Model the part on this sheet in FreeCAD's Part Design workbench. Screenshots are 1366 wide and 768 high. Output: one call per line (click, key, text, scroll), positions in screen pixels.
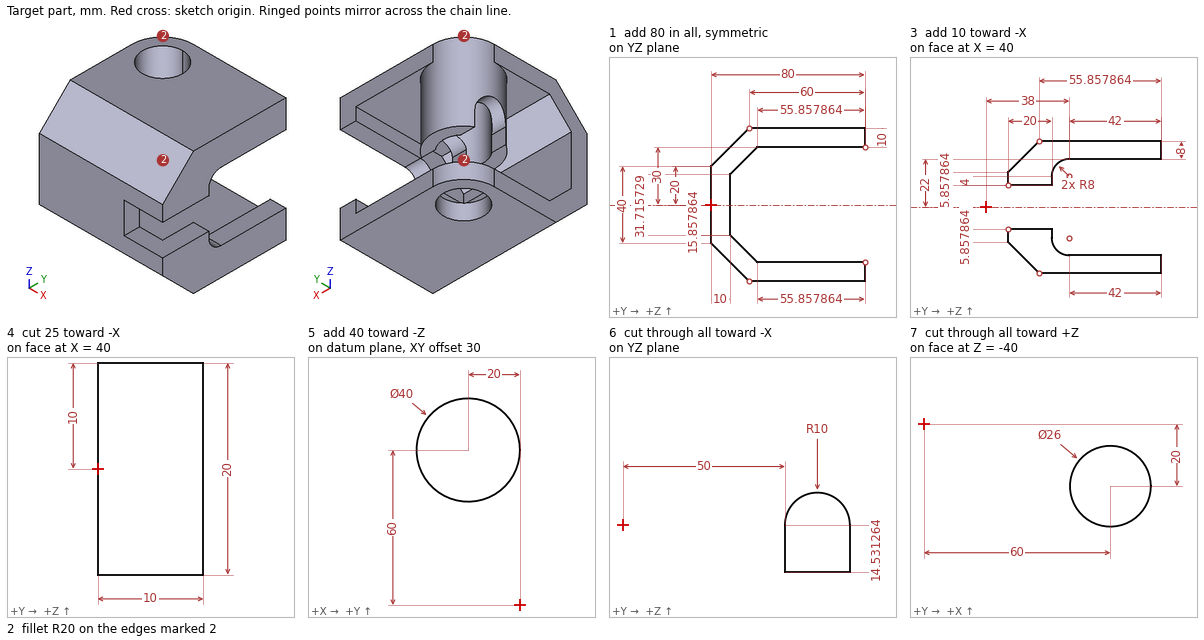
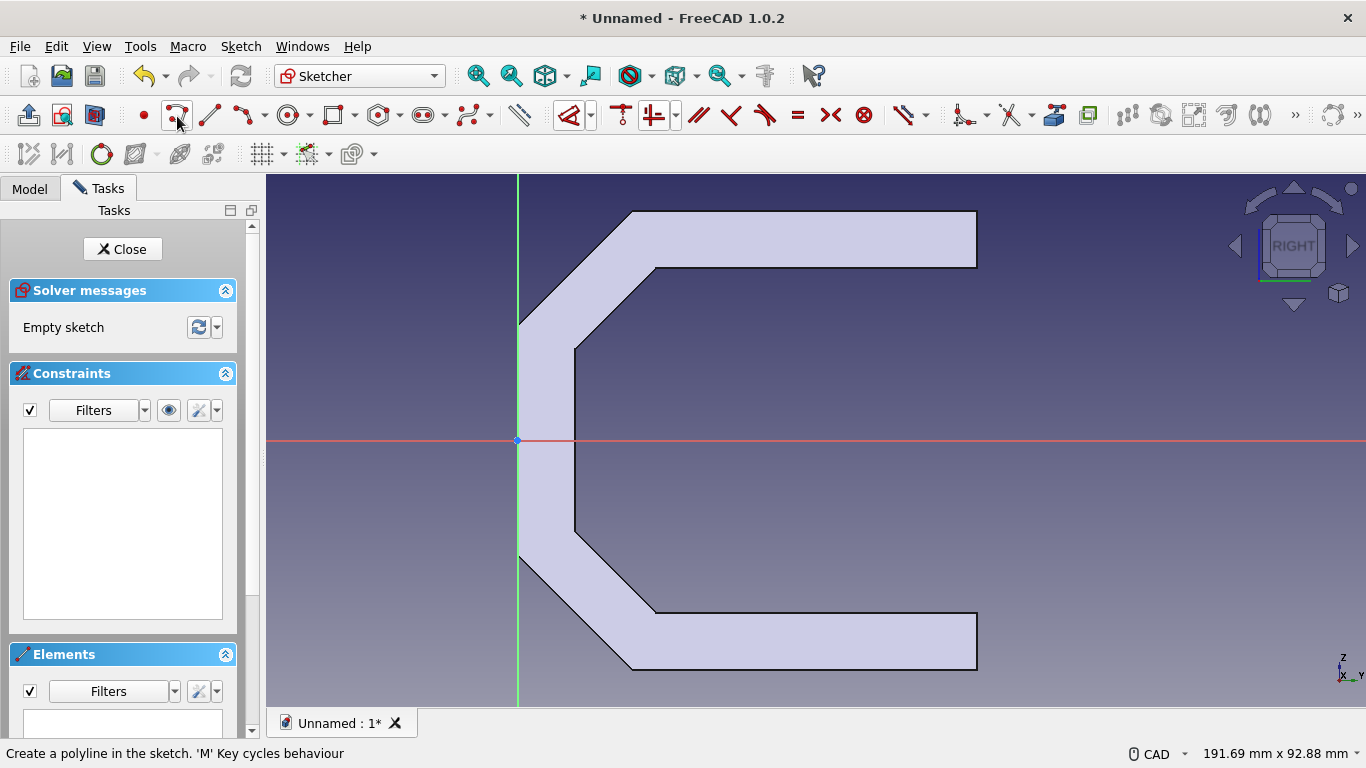
click(736, 314)
click(977, 314)
click(977, 268)
click(656, 268)
click(575, 350)
click(575, 383)
click(690, 383)
click(690, 360)
right_click(690, 360)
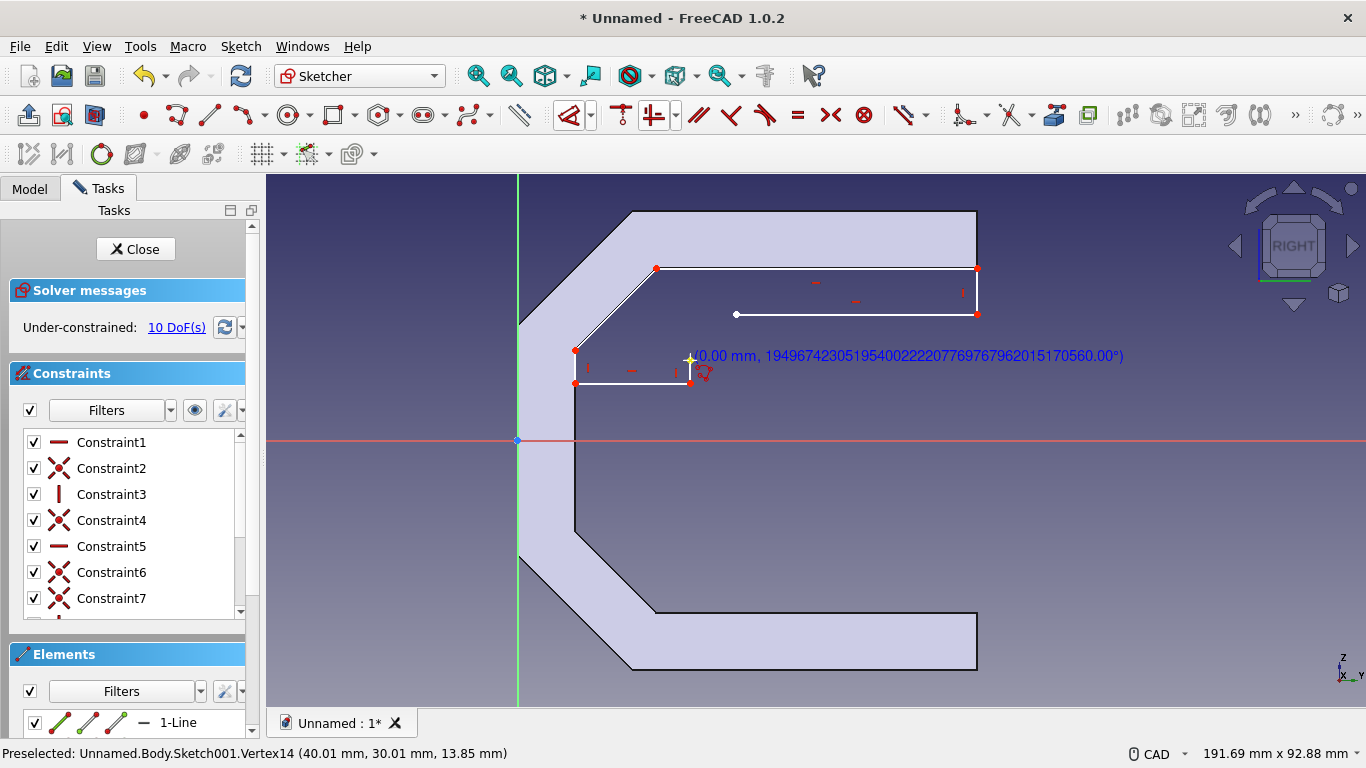
click(242, 116)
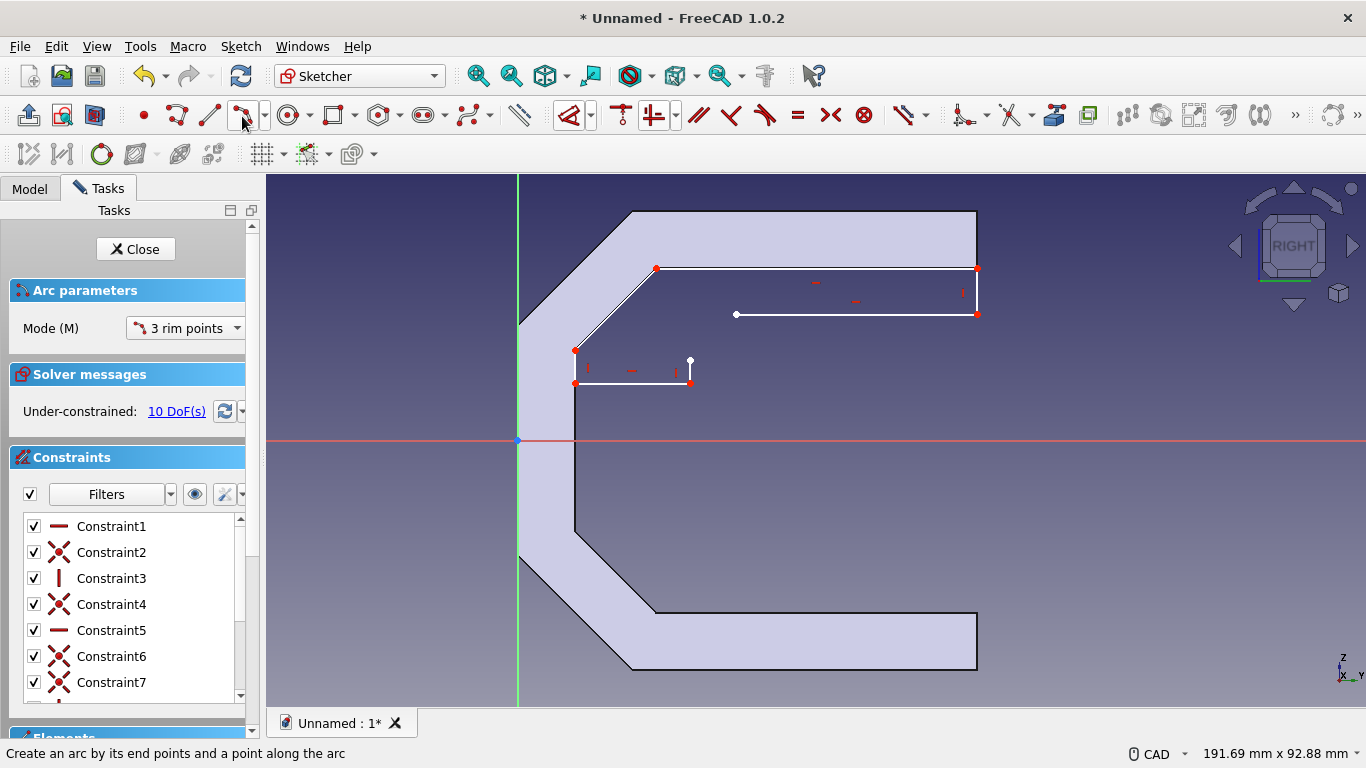
scroll(690, 360, up, 2)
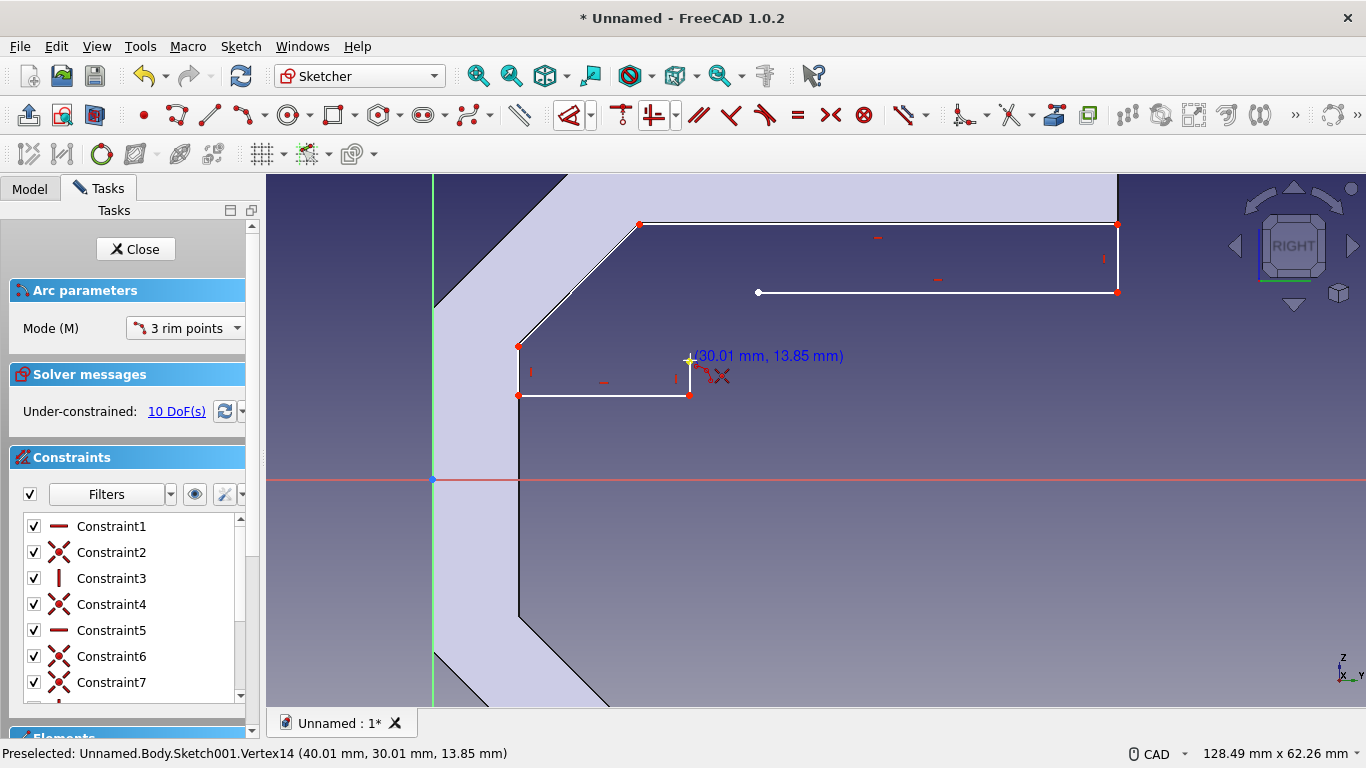
click(690, 361)
click(758, 293)
click(710, 312)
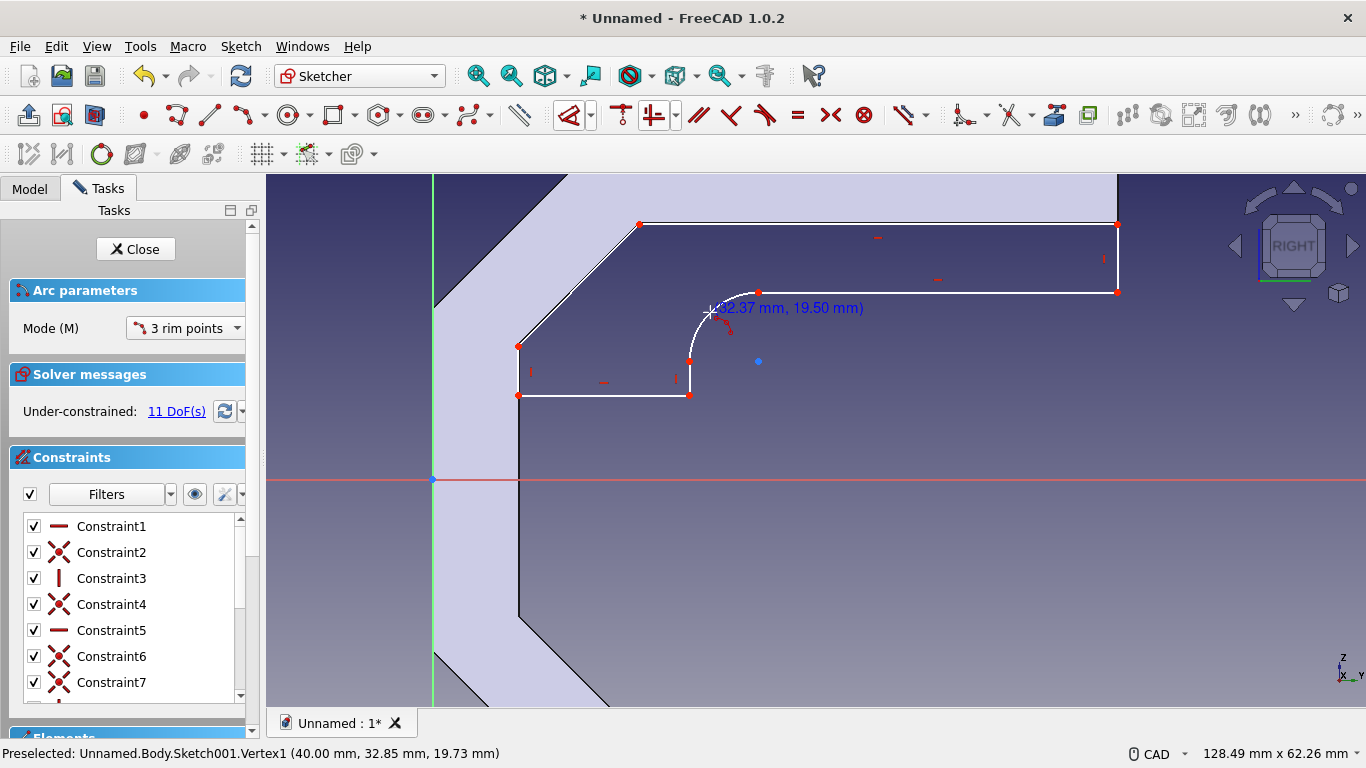
key(g)
key(m)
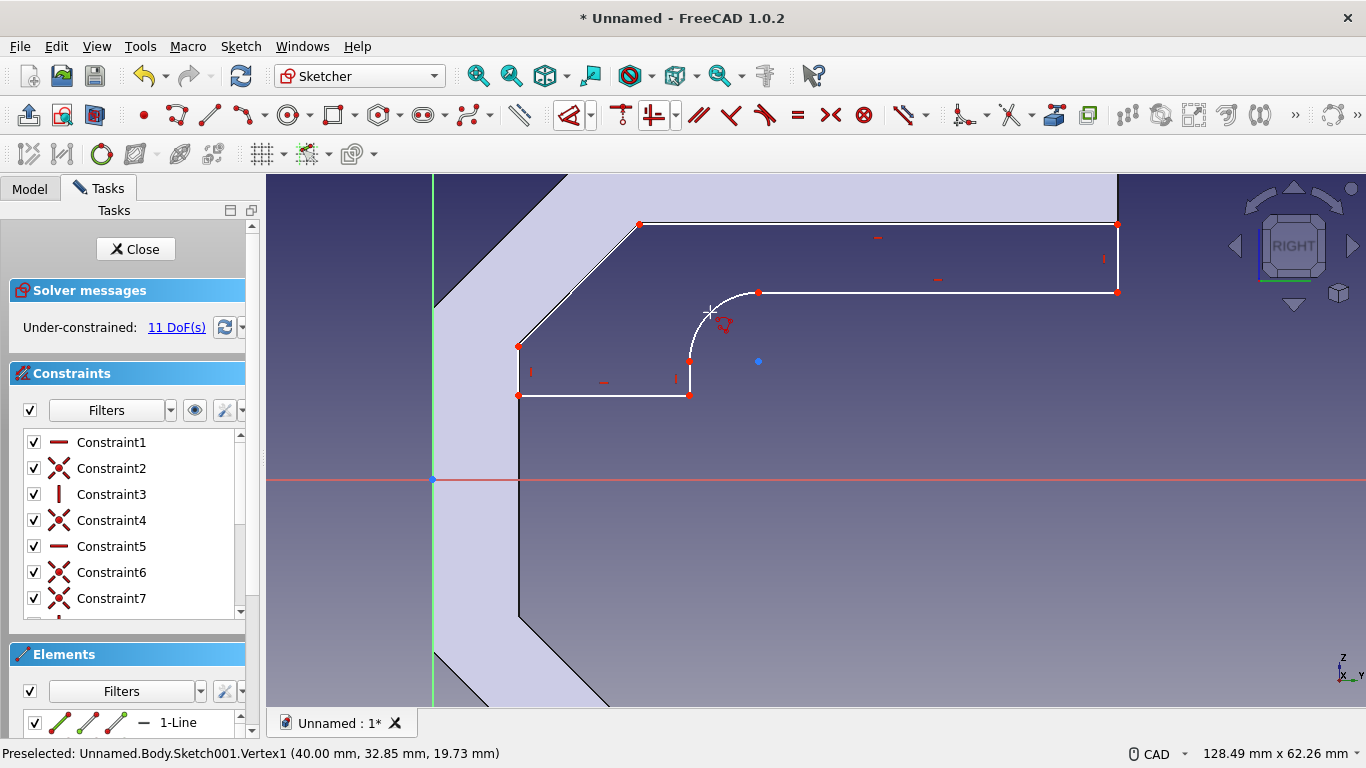
click(690, 600)
click(690, 566)
click(519, 566)
click(519, 616)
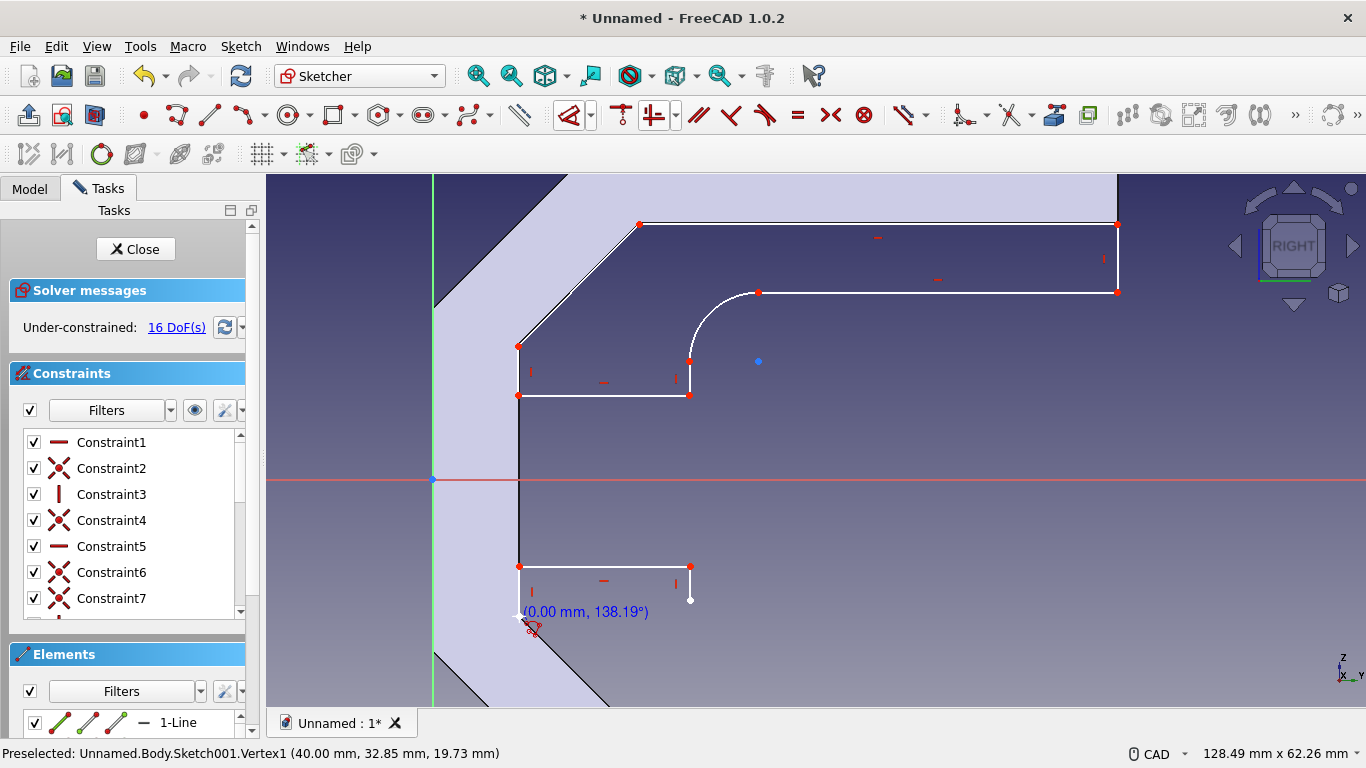
scroll(691, 360, down, 2)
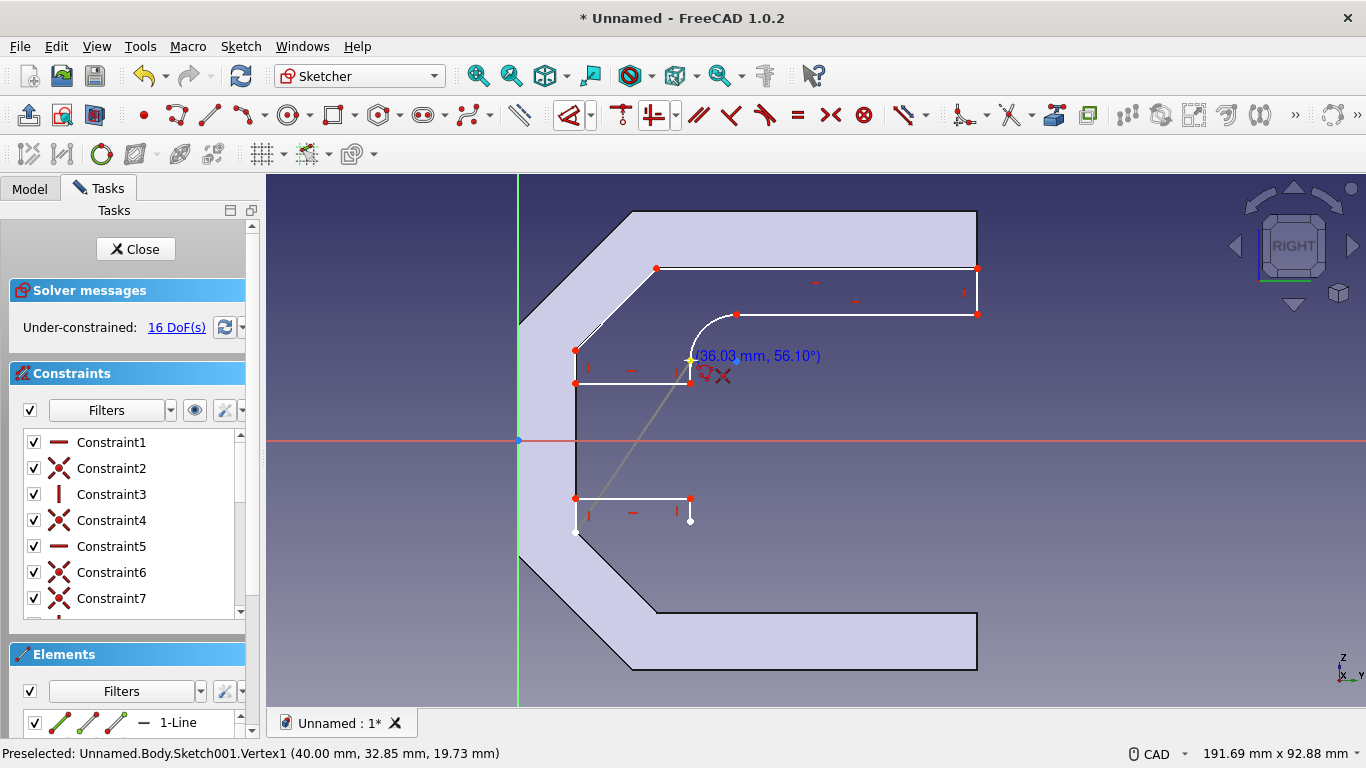
click(657, 613)
click(977, 613)
click(977, 567)
click(736, 567)
right_click(736, 567)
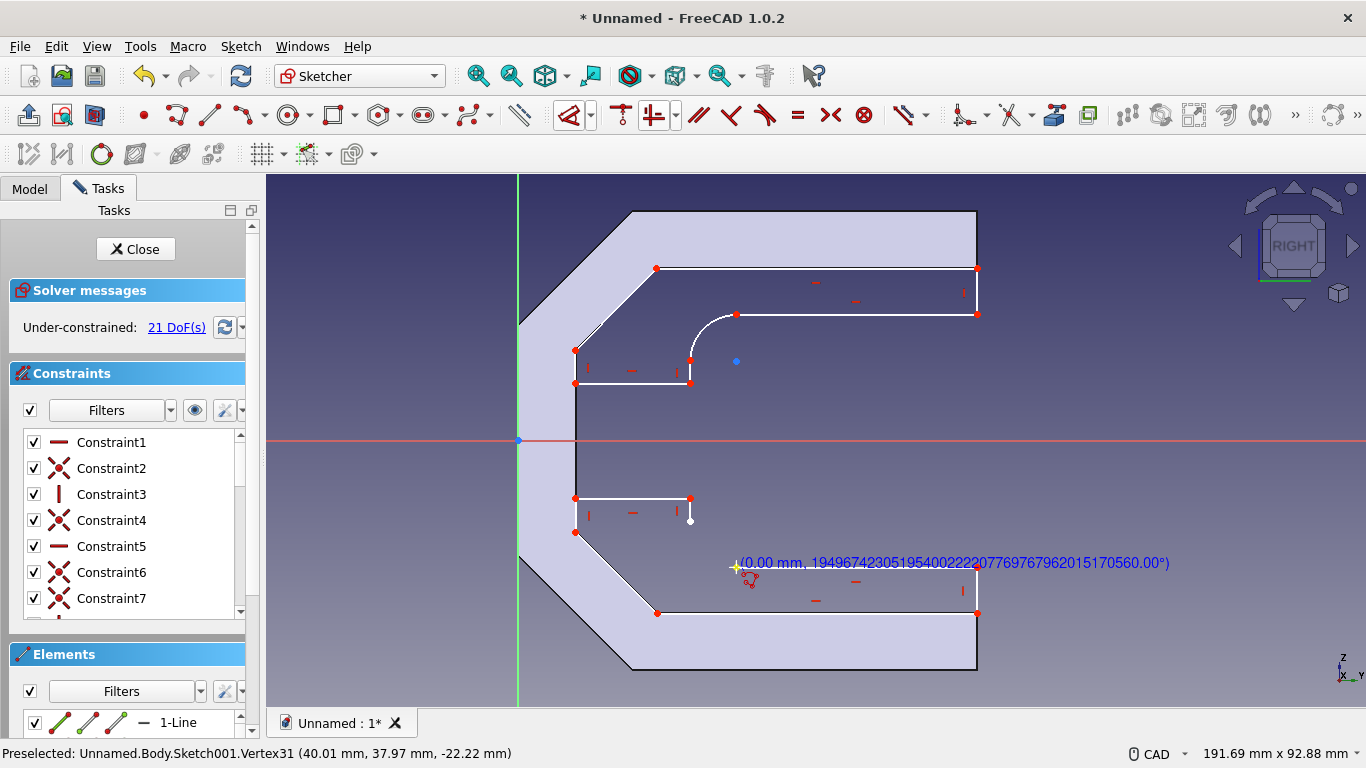
click(242, 116)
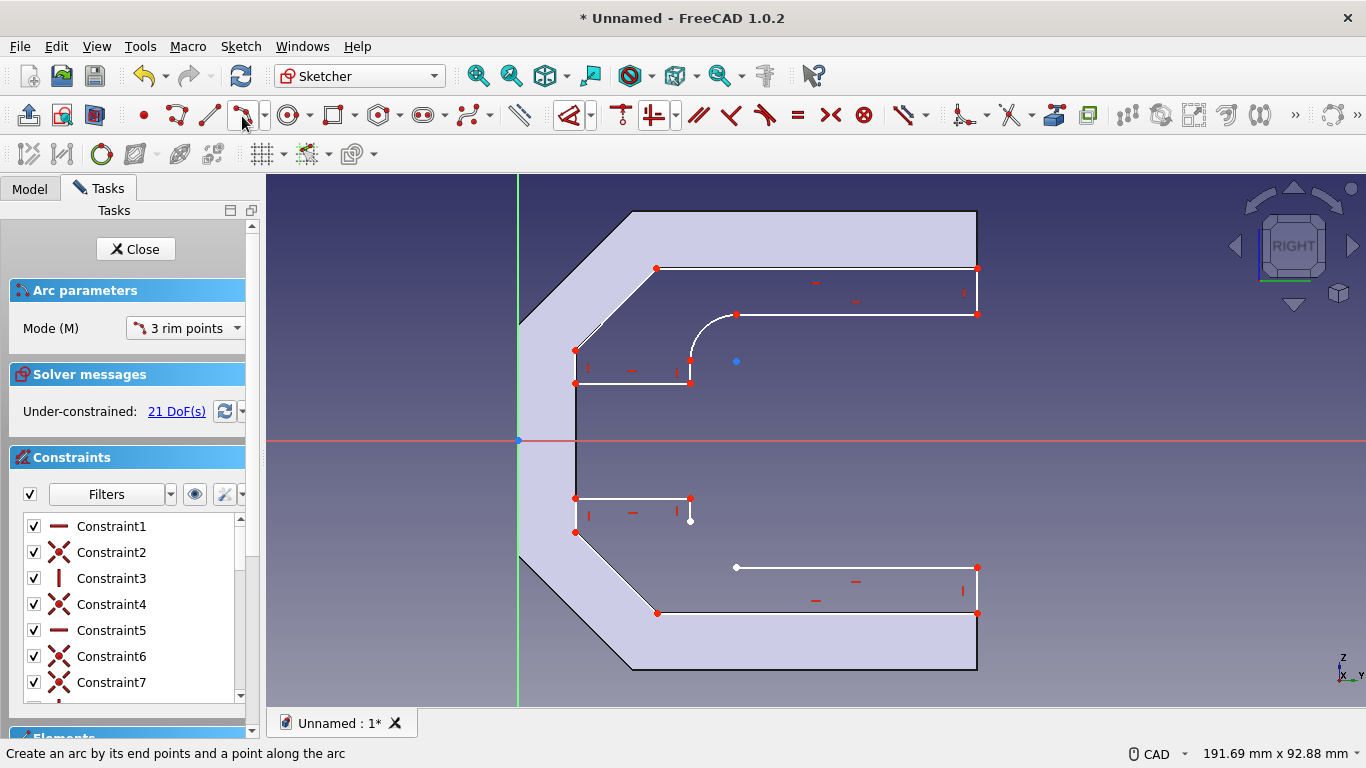
click(736, 568)